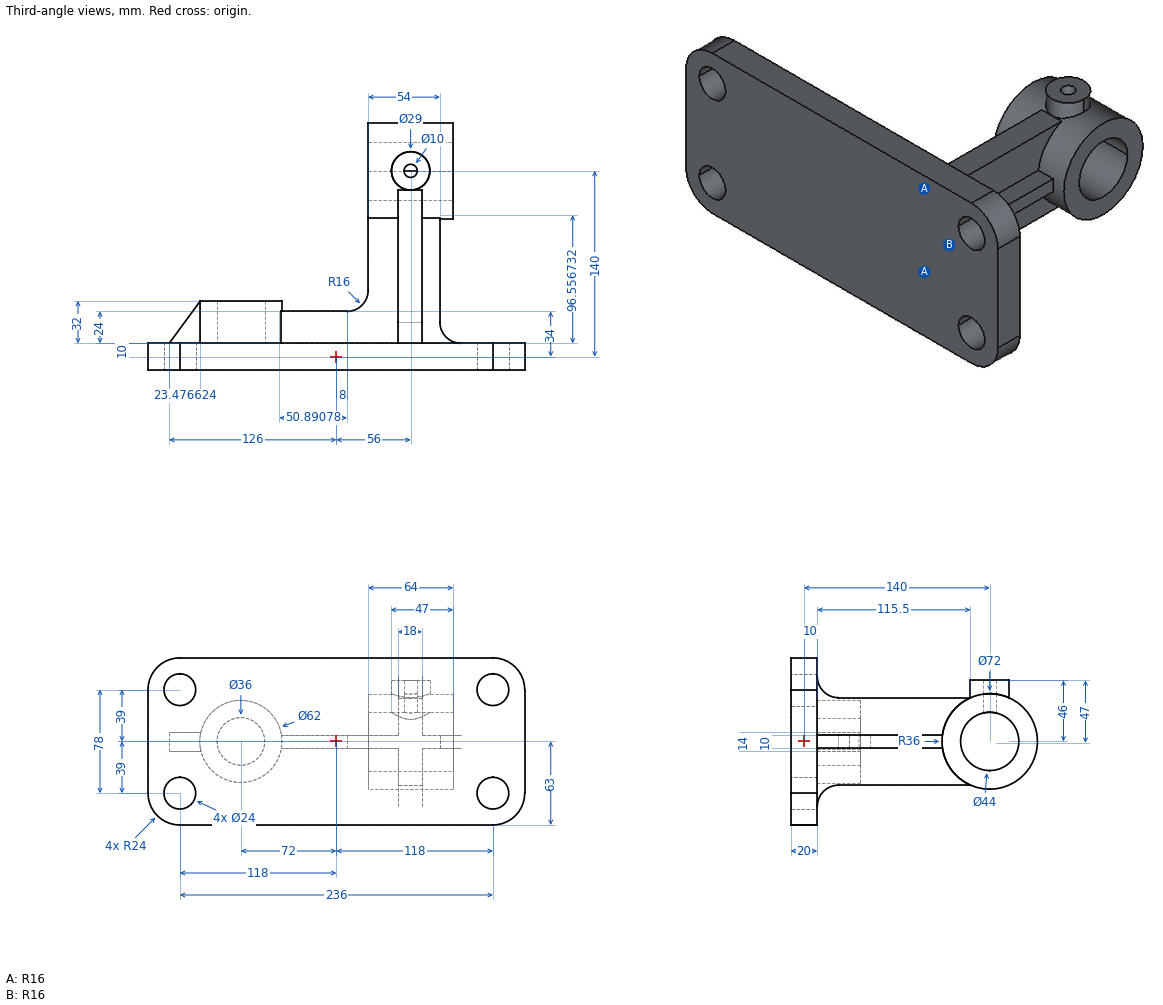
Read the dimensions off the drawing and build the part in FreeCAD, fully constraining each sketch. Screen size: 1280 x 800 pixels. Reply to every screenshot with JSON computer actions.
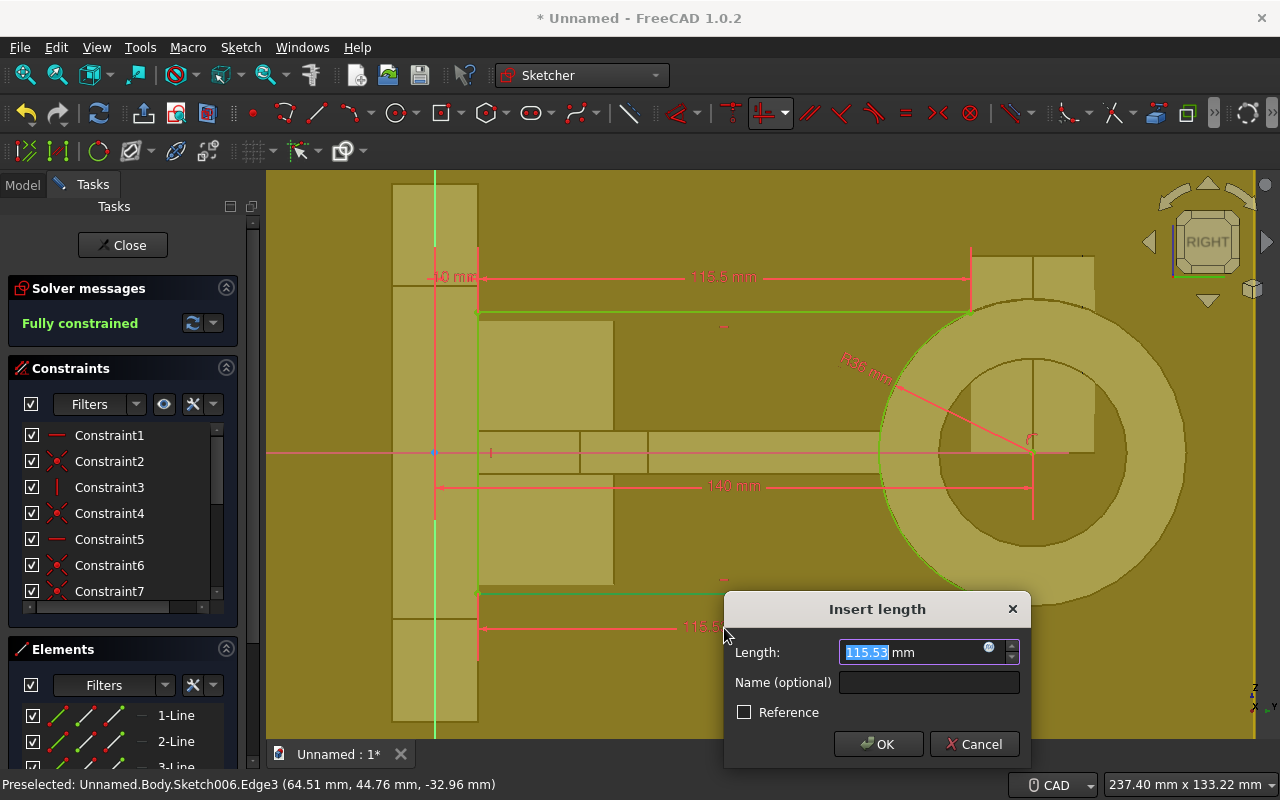
{"action": "type", "text": "115.5"}
{"action": "key", "text": "Return"}
{"action": "key", "text": "Escape"}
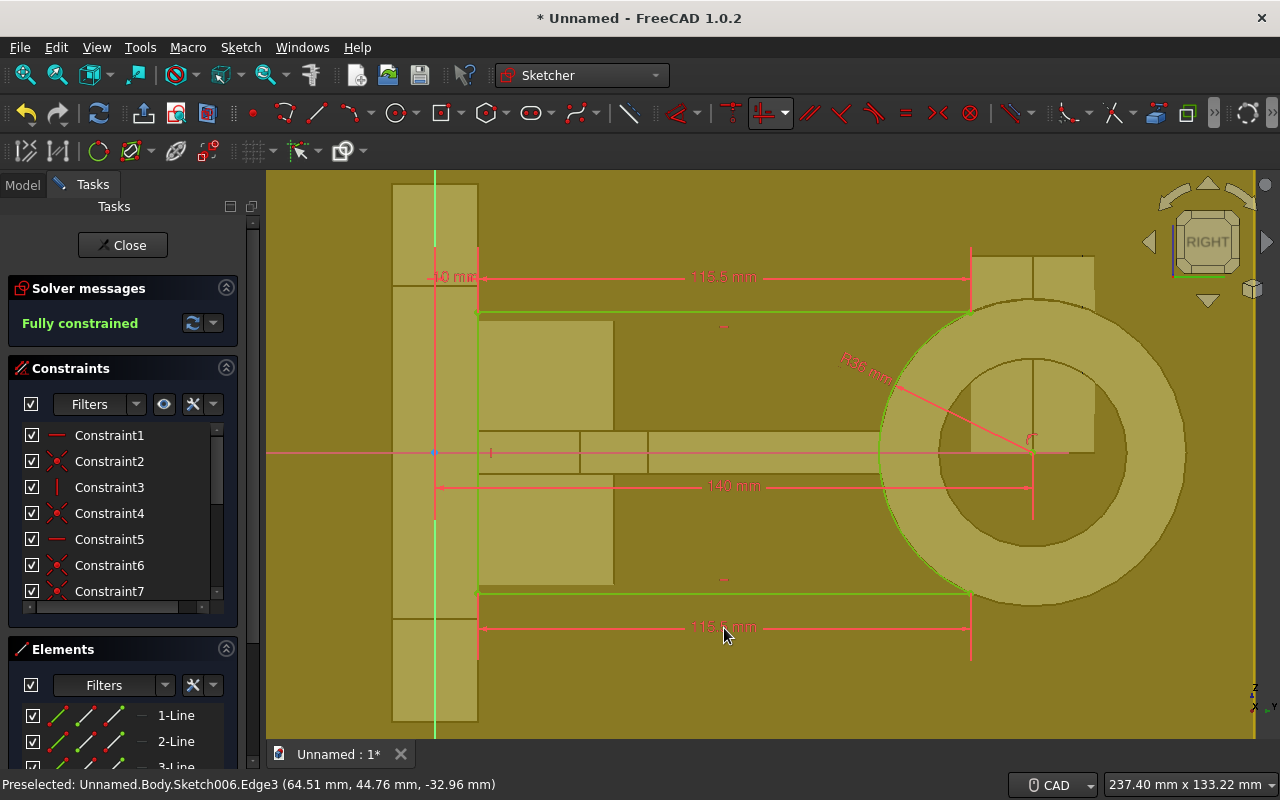
{"action": "left_click", "coordinate": [123, 245]}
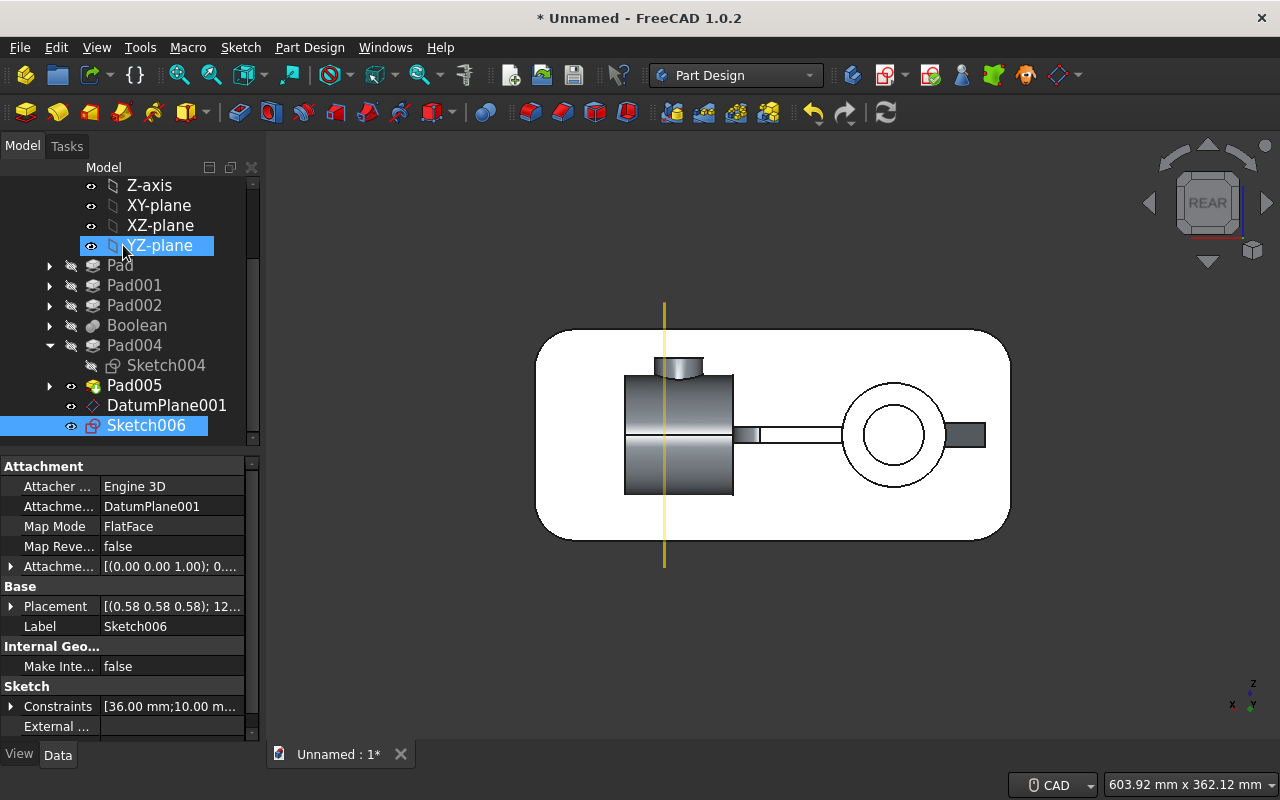
{"action": "left_click", "coordinate": [26, 112]}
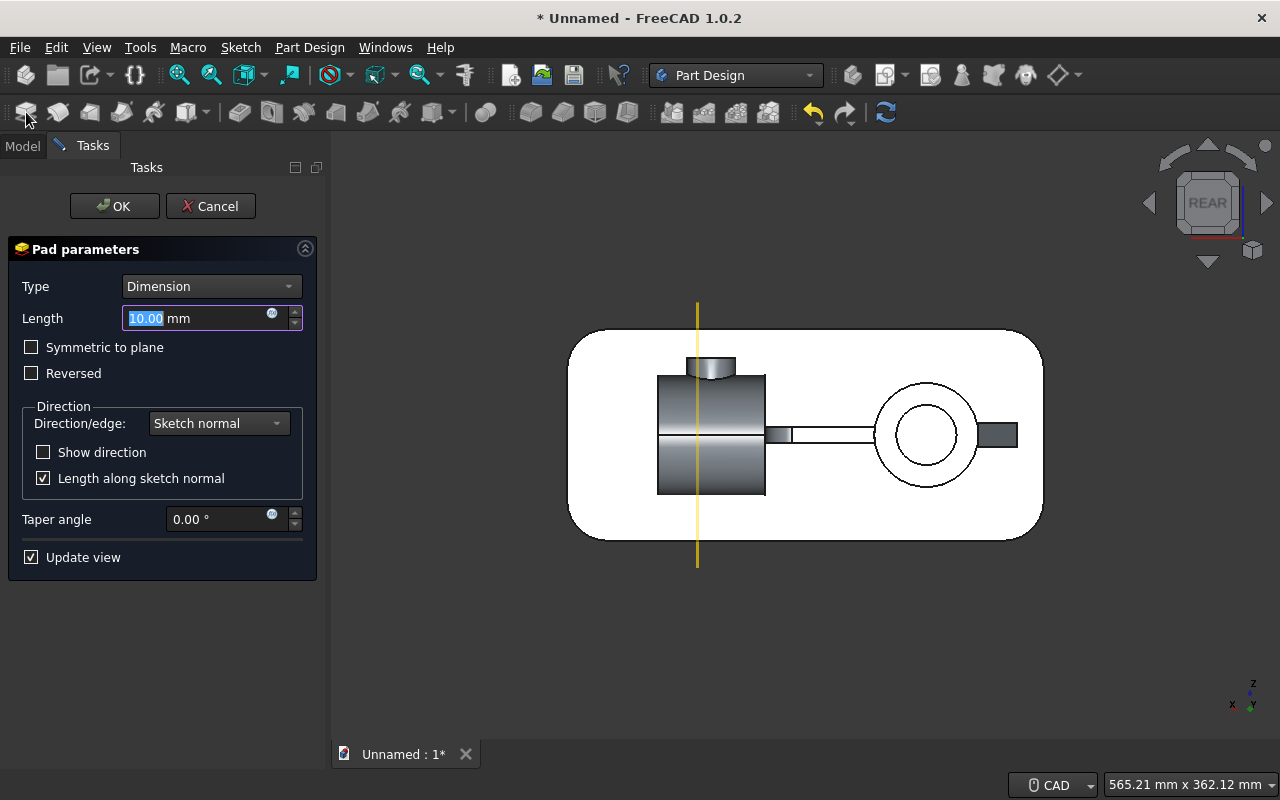
{"action": "type", "text": "18"}
{"action": "key", "text": "Tab"}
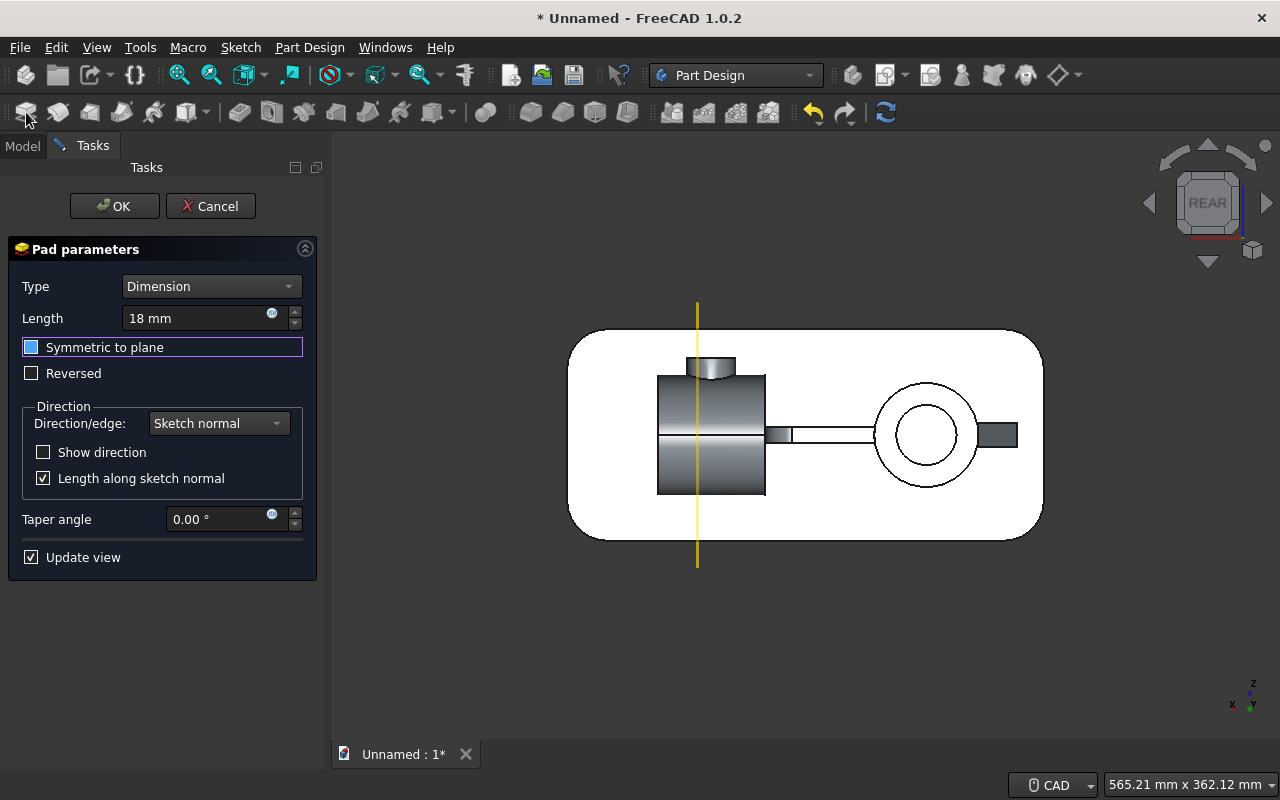
{"action": "left_click", "coordinate": [30, 373]}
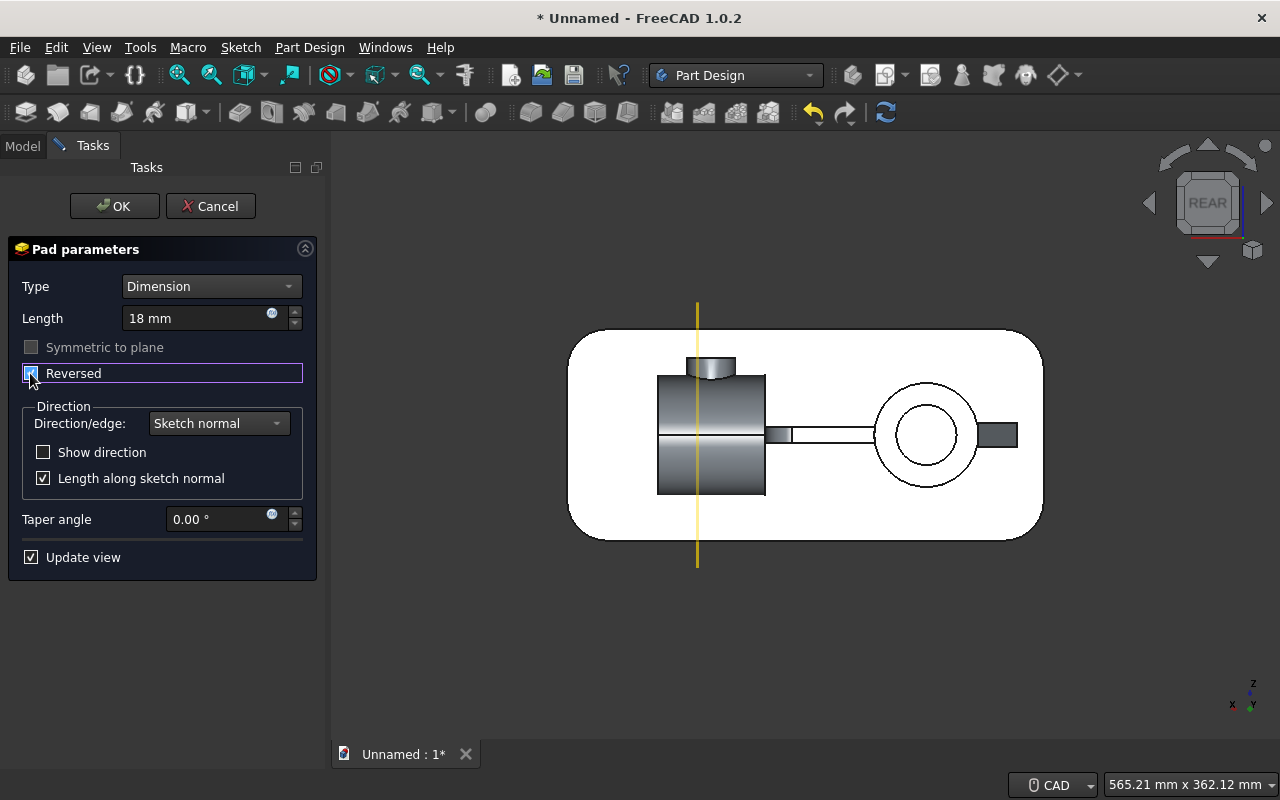
{"action": "left_click", "coordinate": [115, 206]}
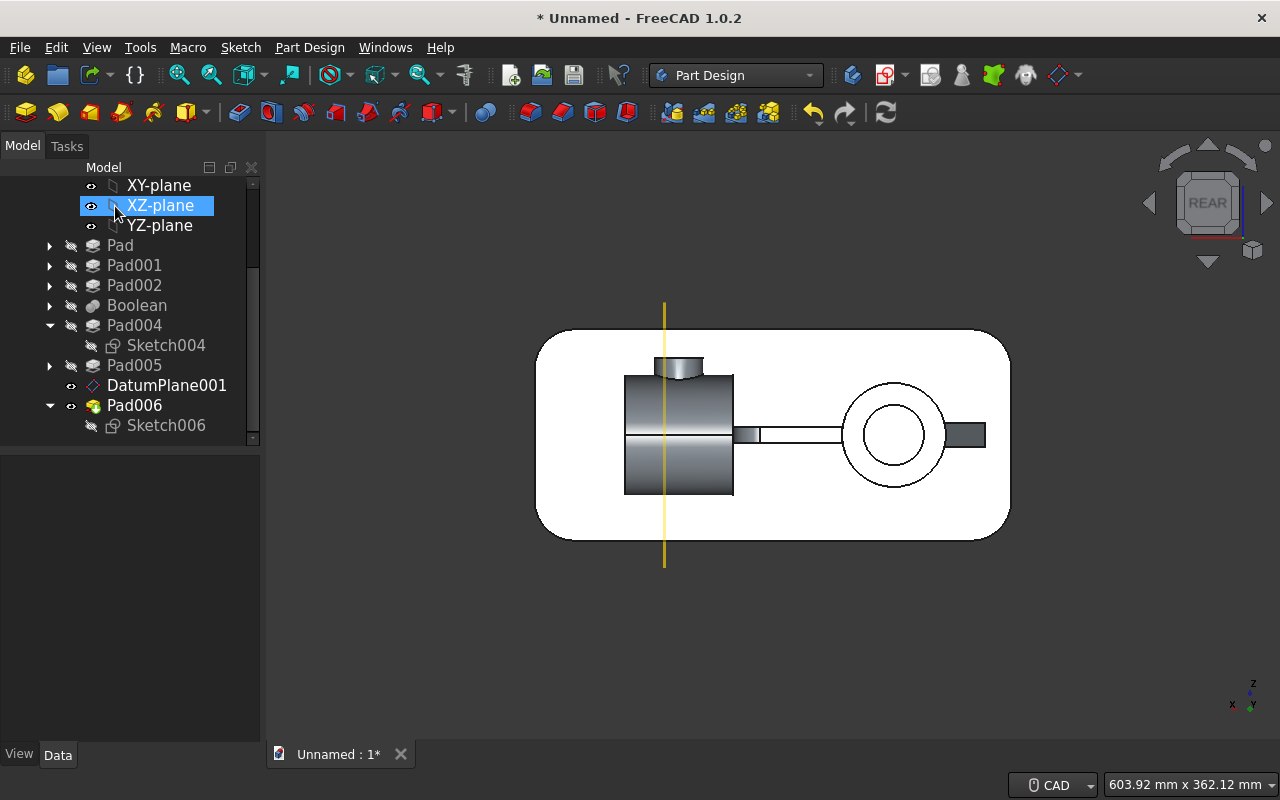
{"action": "left_click", "coordinate": [116, 386]}
{"action": "key", "text": "space"}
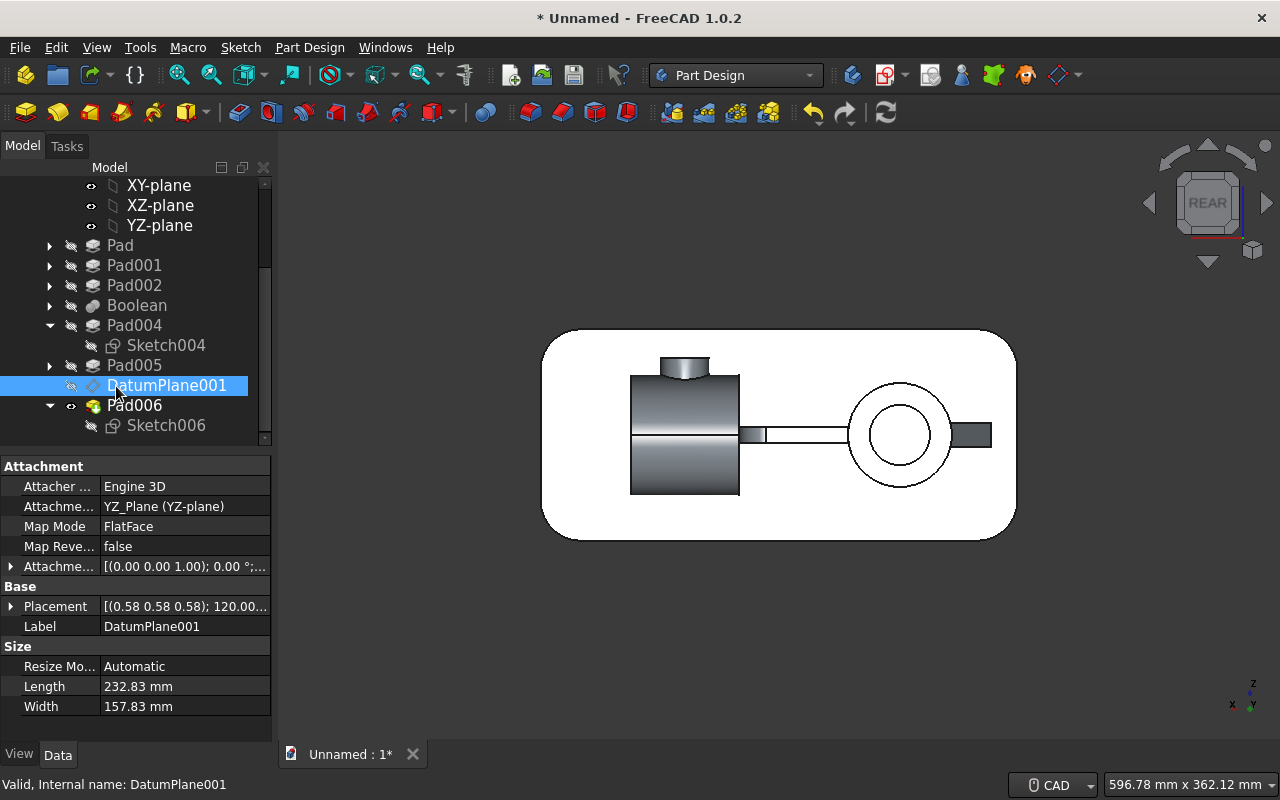
{"action": "key", "text": "0"}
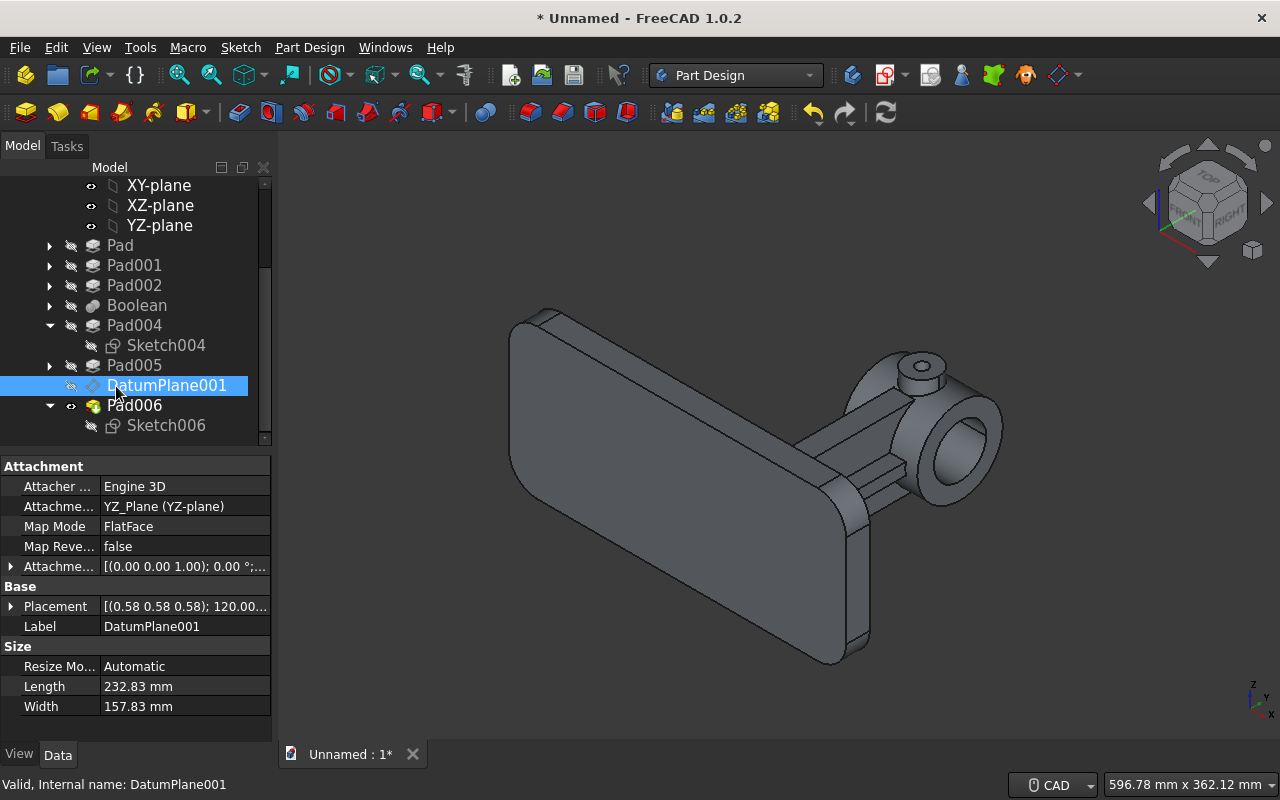
{"action": "key", "text": "2"}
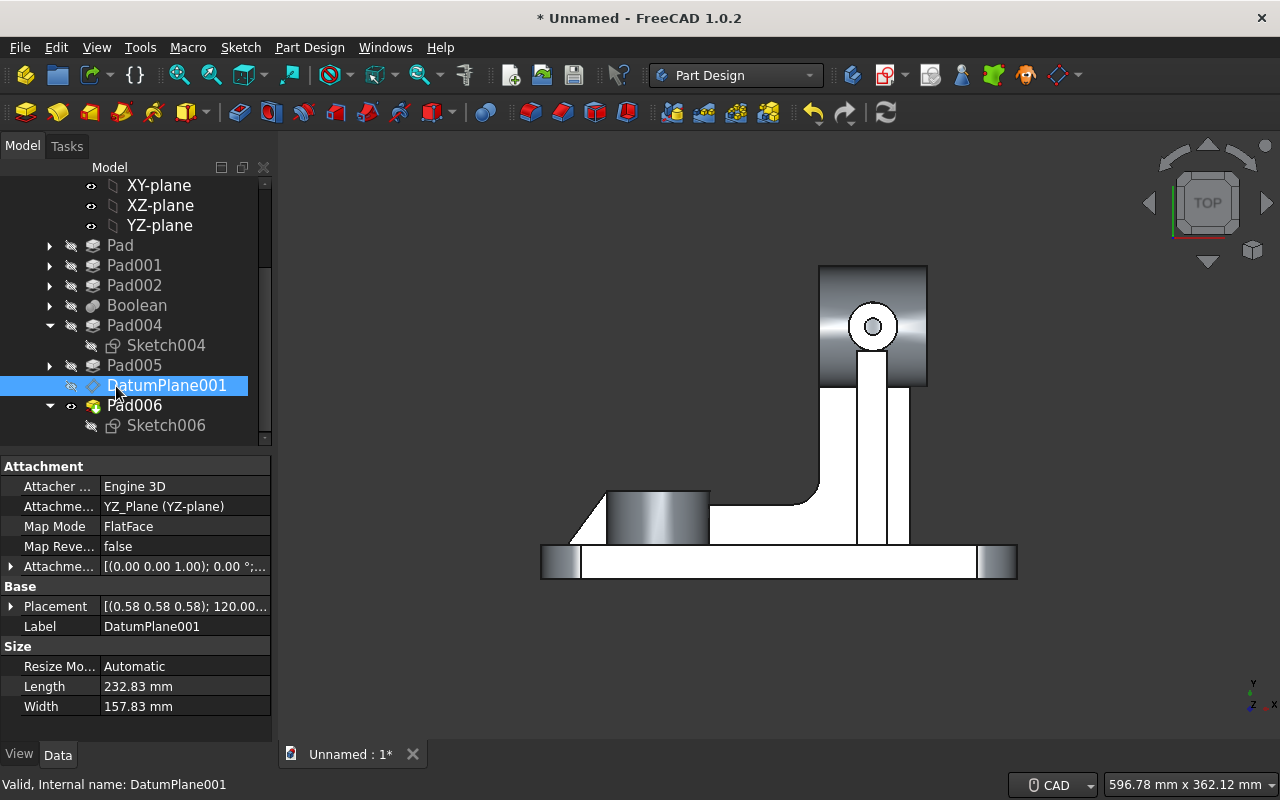
{"action": "key", "text": "1"}